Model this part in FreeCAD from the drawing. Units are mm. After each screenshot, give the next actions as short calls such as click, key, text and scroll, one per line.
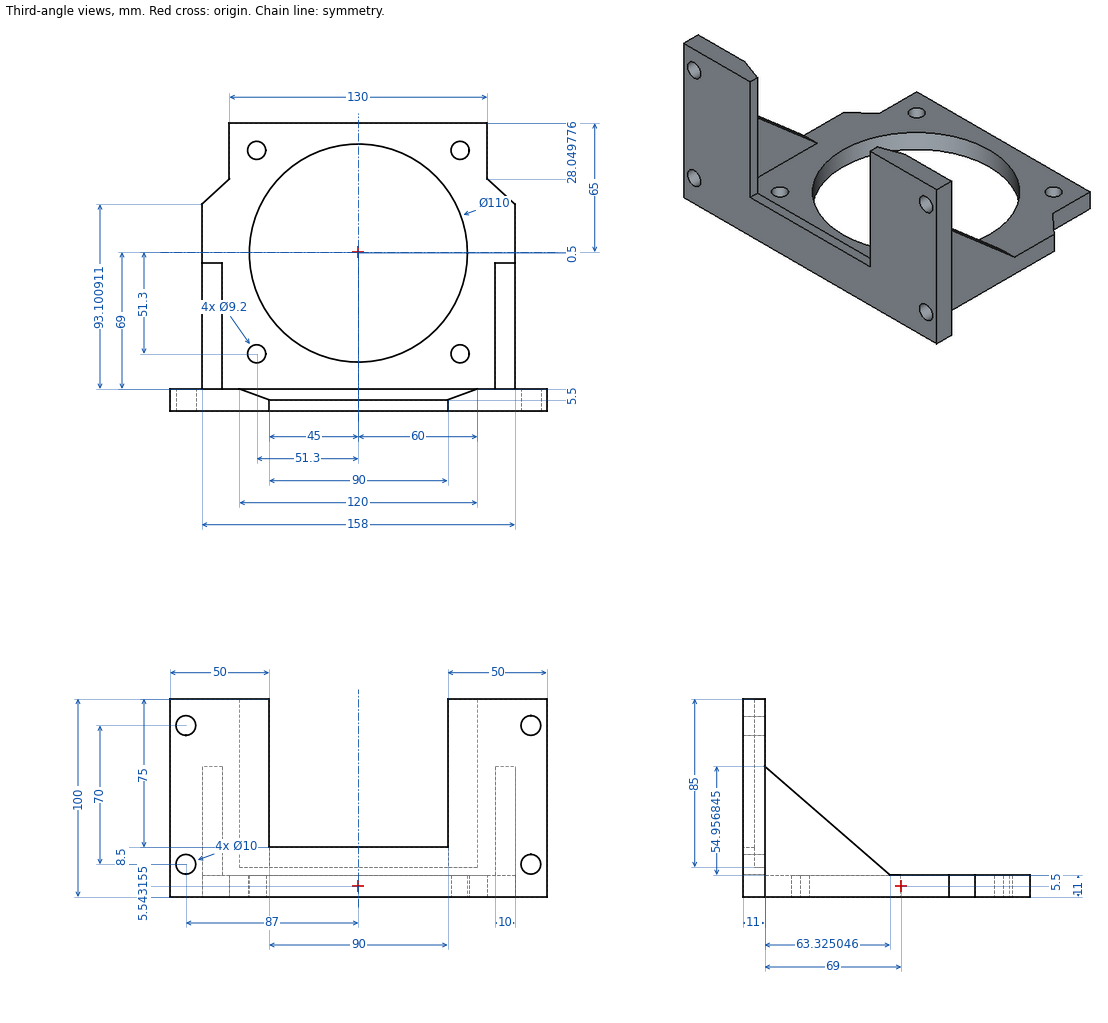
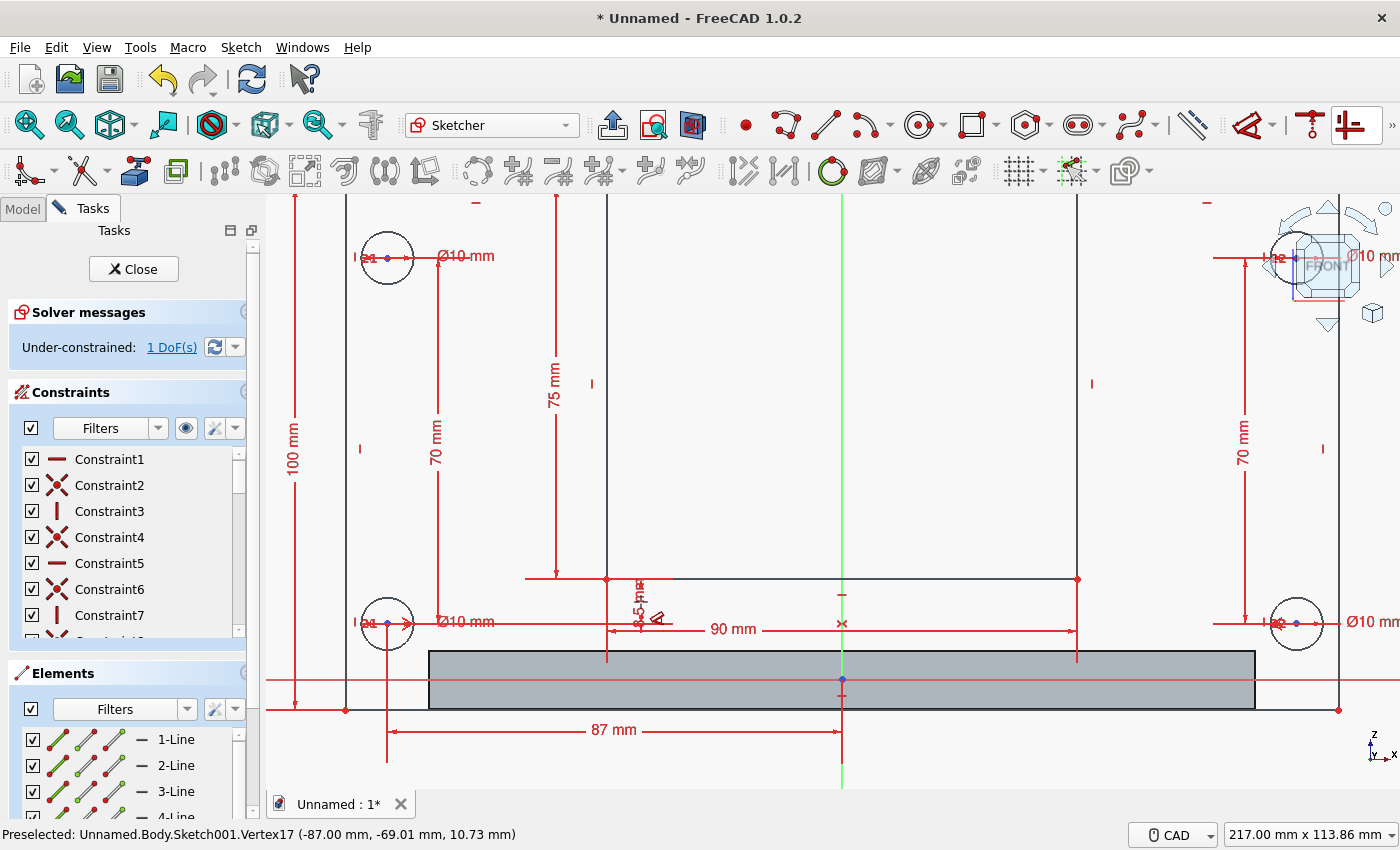
scroll(346, 710, up, 2)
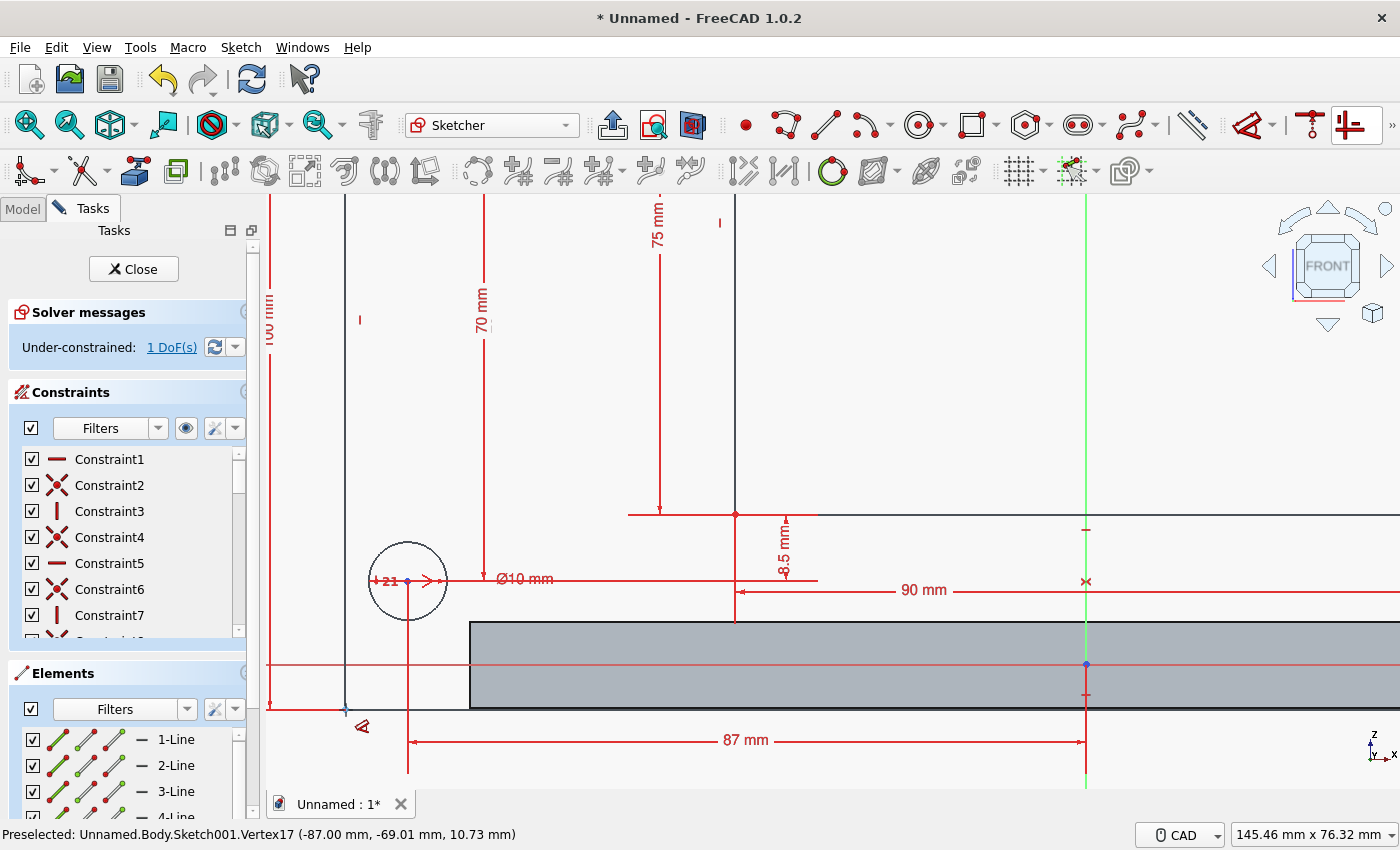
click(345, 710)
click(311, 687)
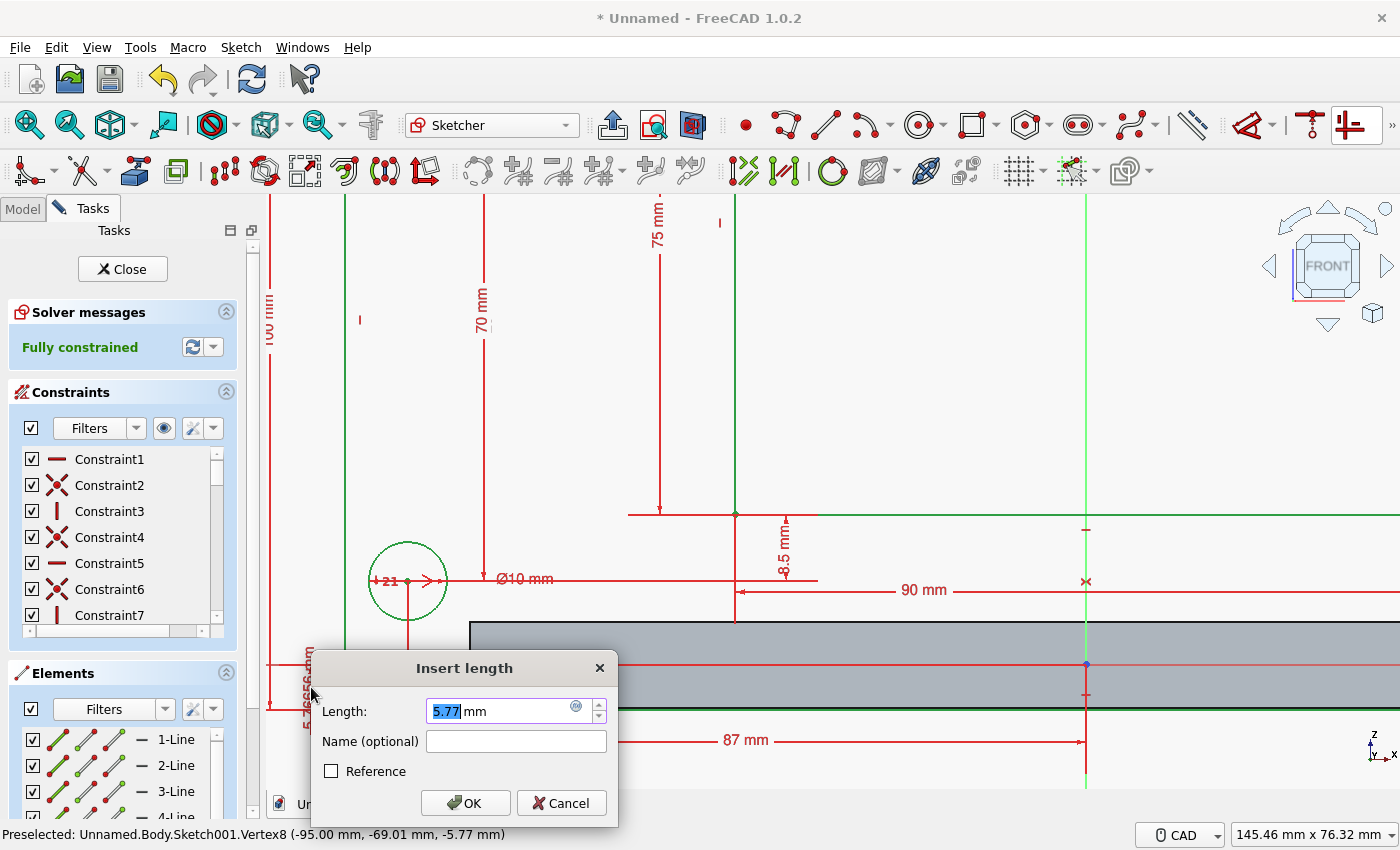
text(5.543155)
key(Return)
key(Escape)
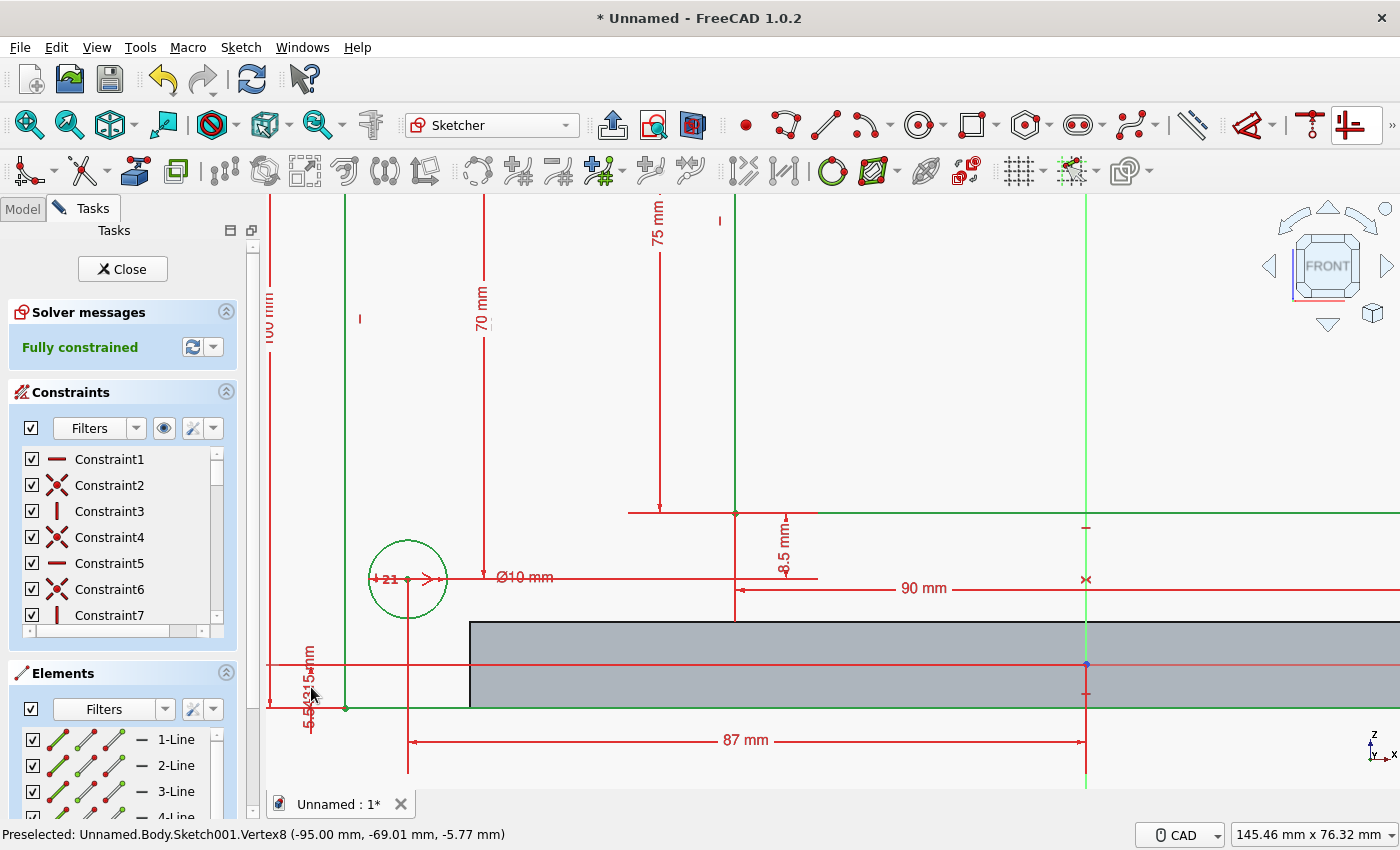
click(123, 269)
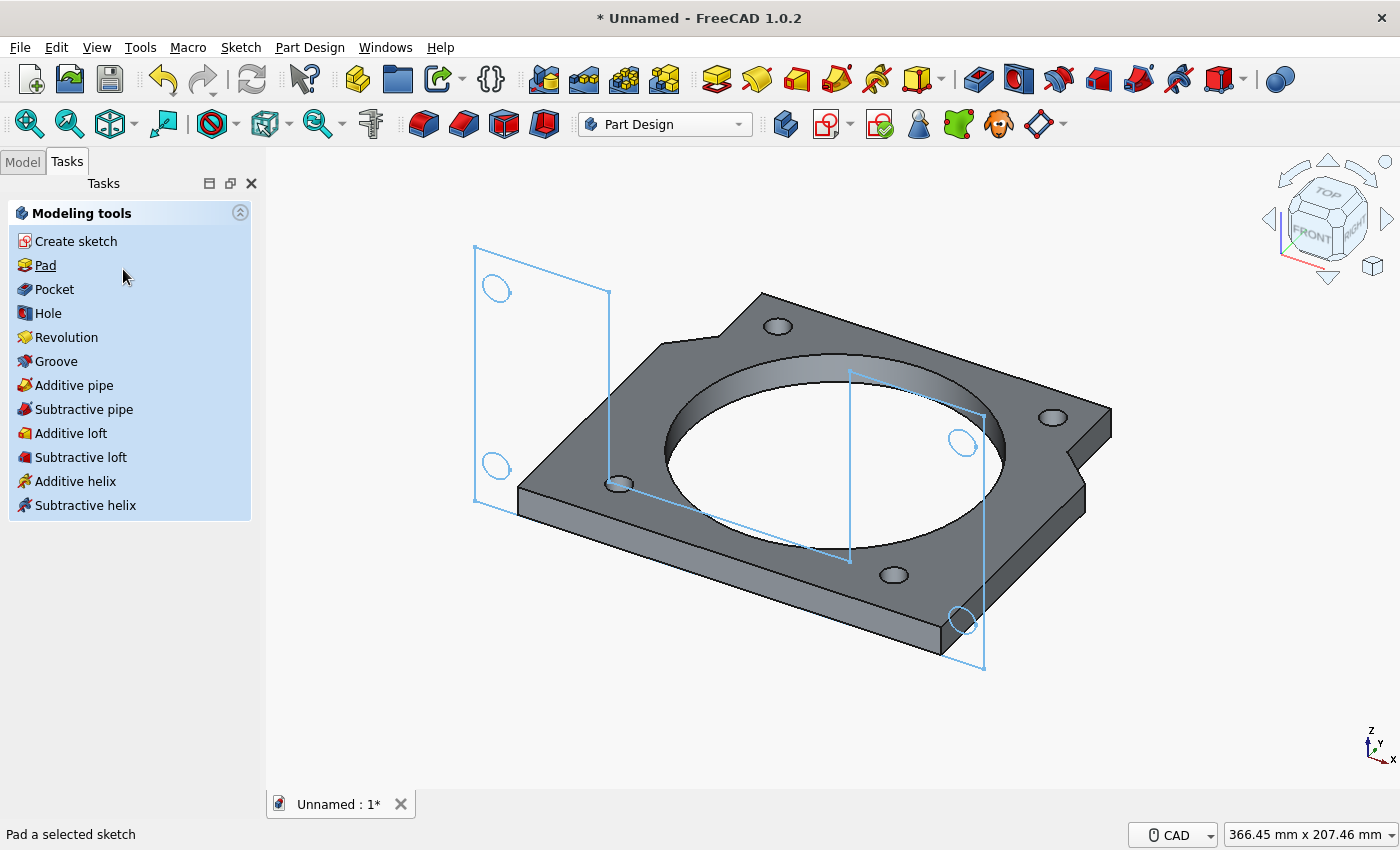
click(718, 80)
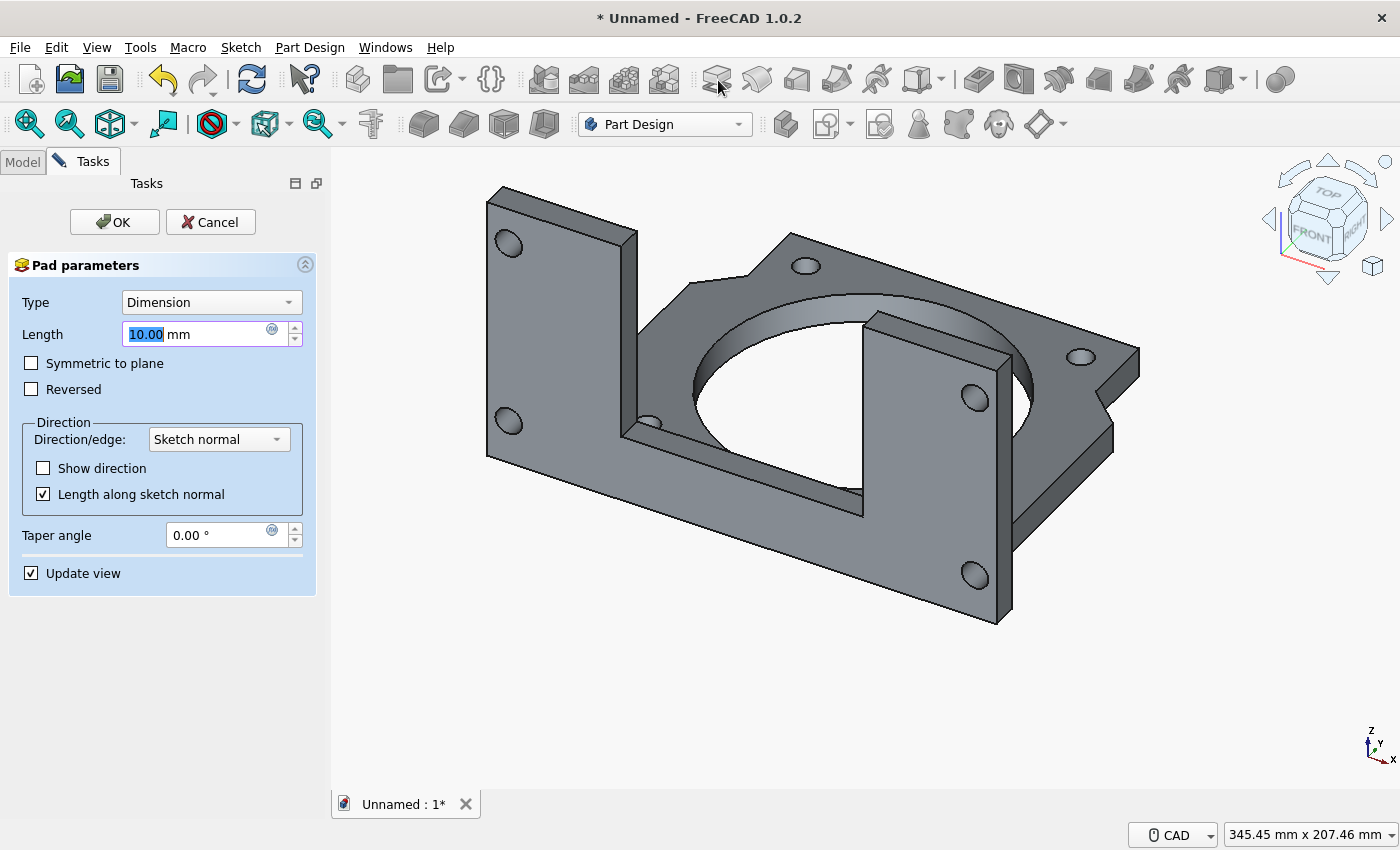
text(11)
key(Tab)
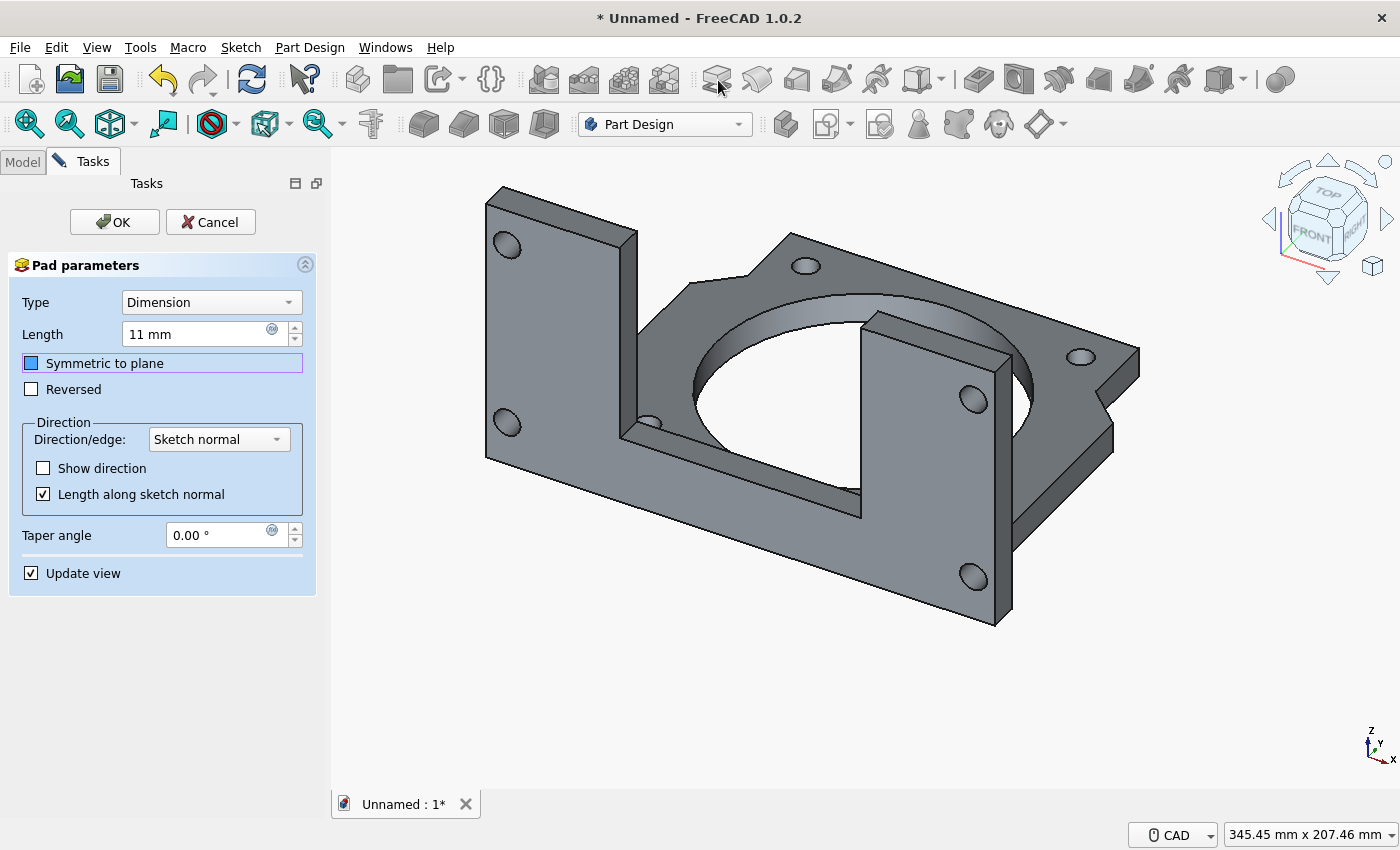
click(115, 222)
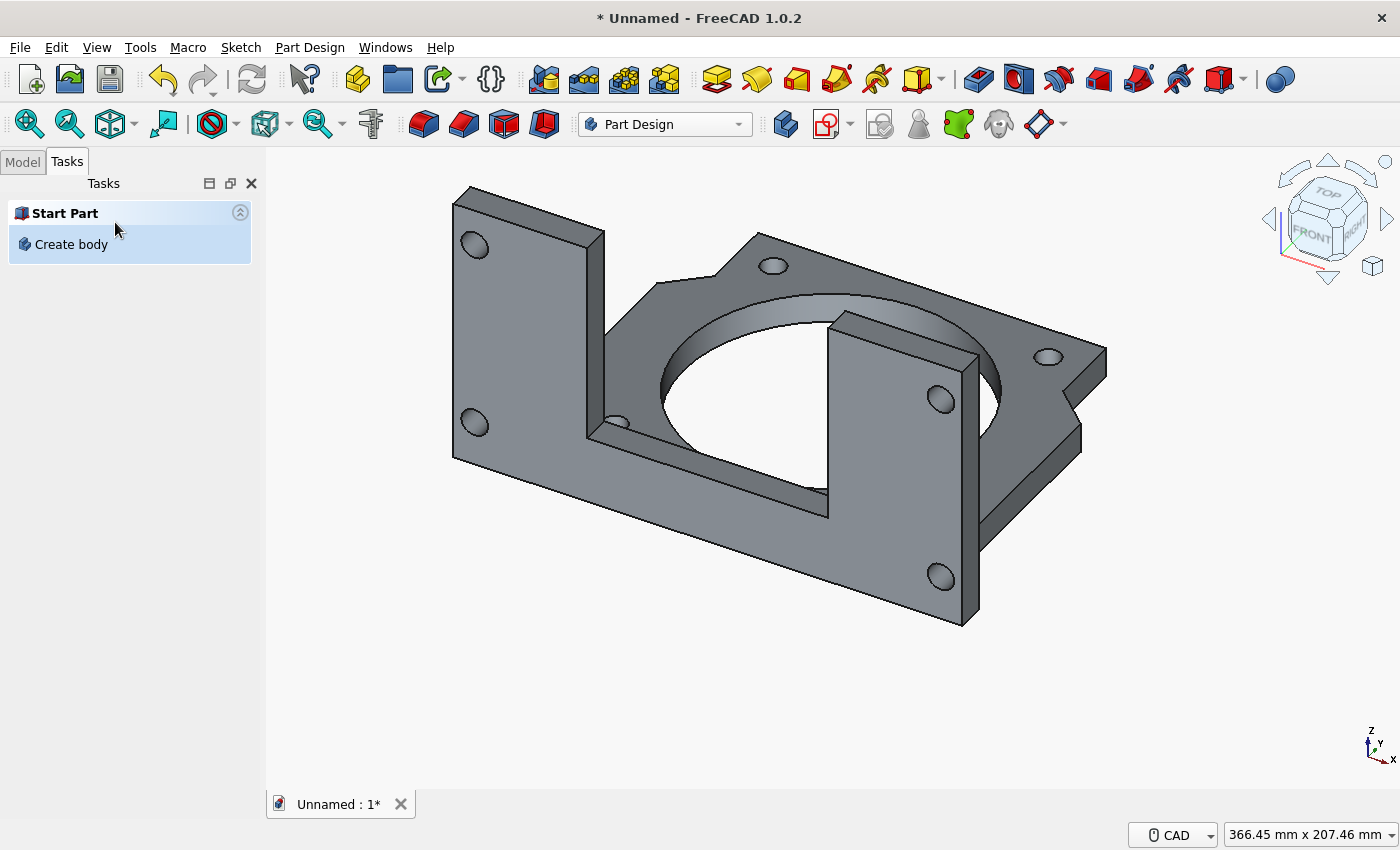
click(30, 124)